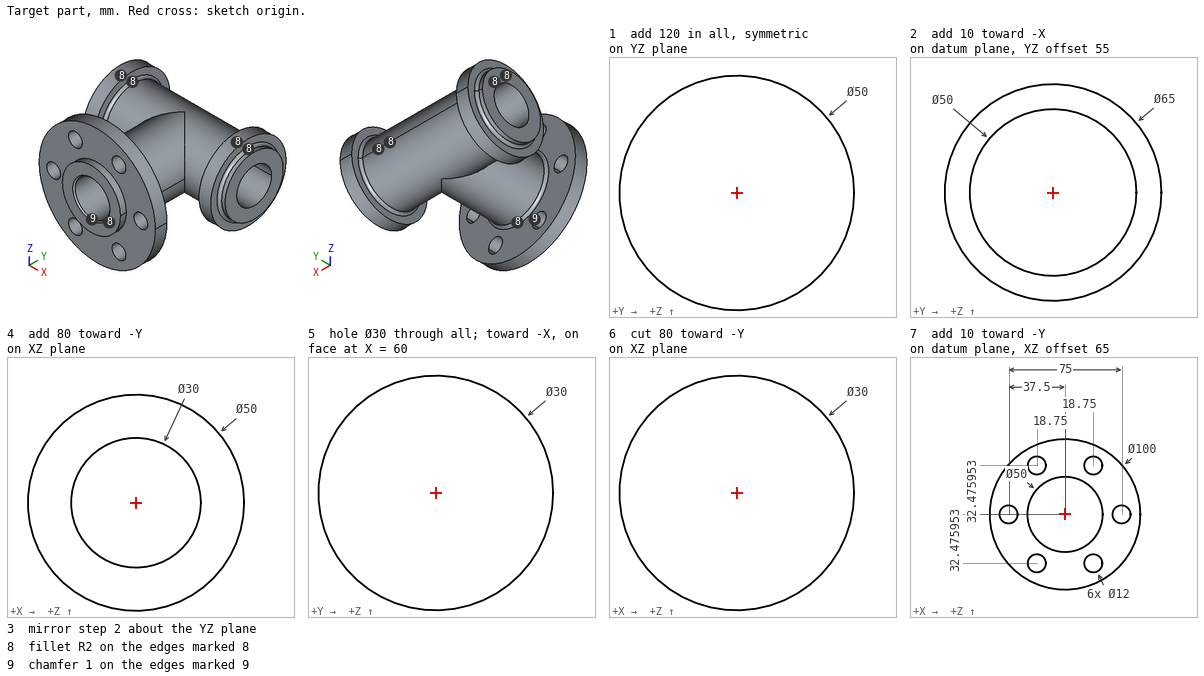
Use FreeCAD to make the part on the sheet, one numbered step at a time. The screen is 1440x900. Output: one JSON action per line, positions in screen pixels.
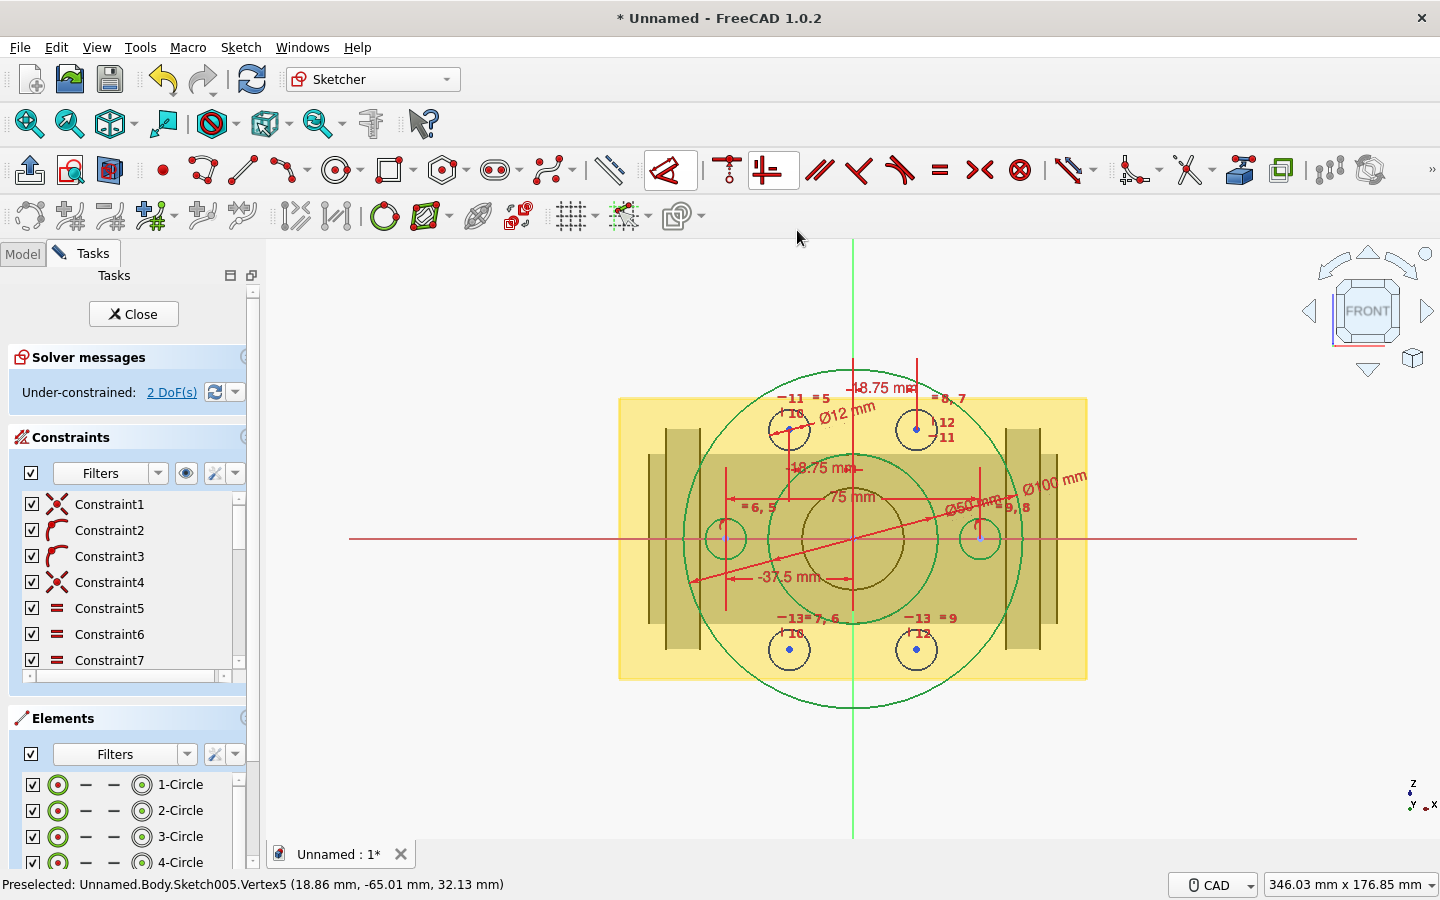
{"action": "left_click", "coordinate": [789, 430]}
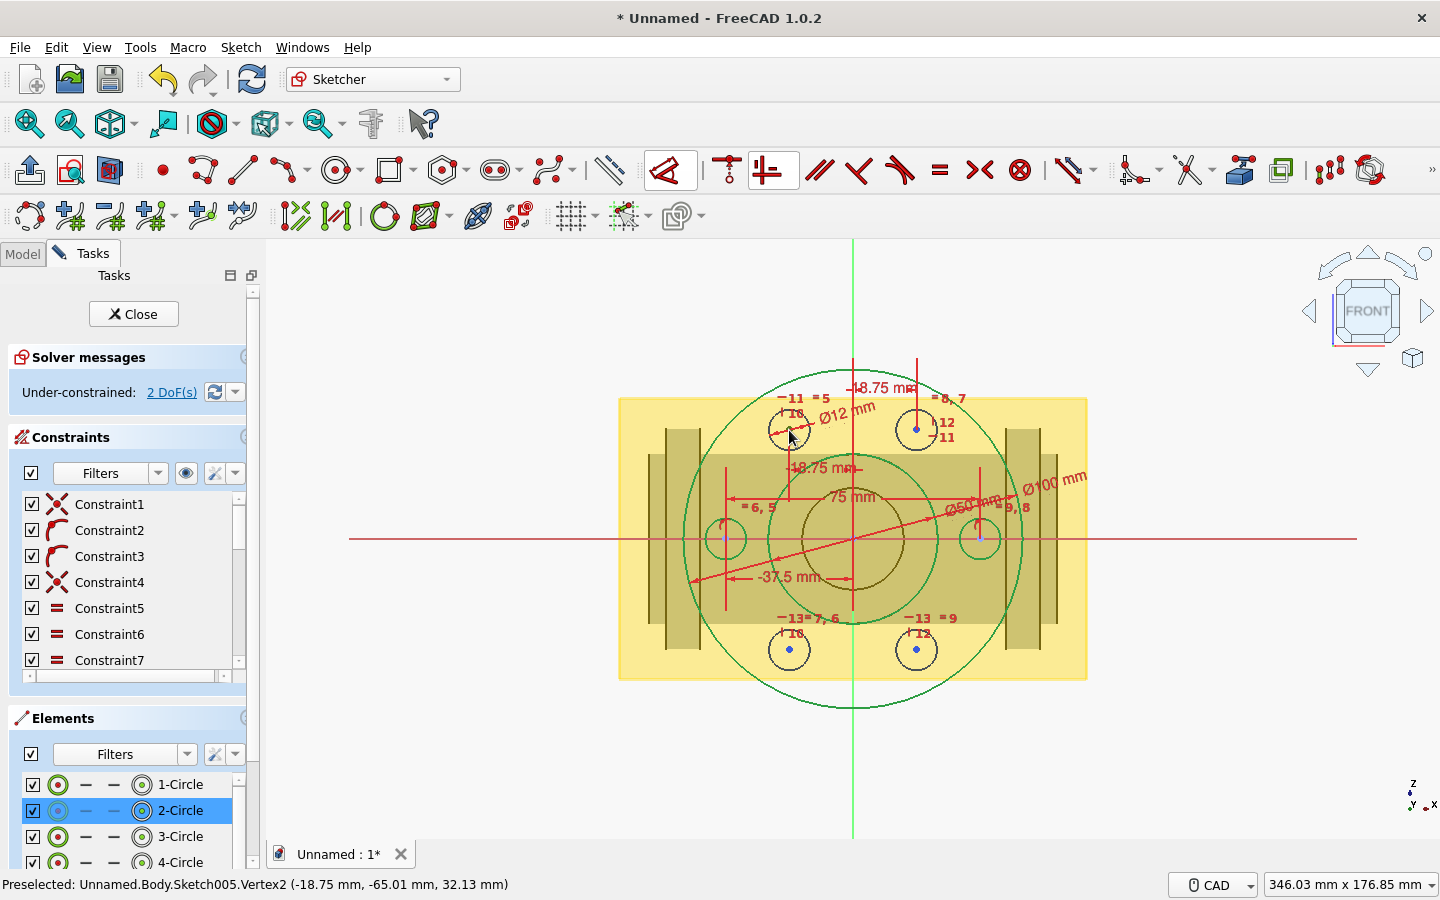
{"action": "key", "text": "i"}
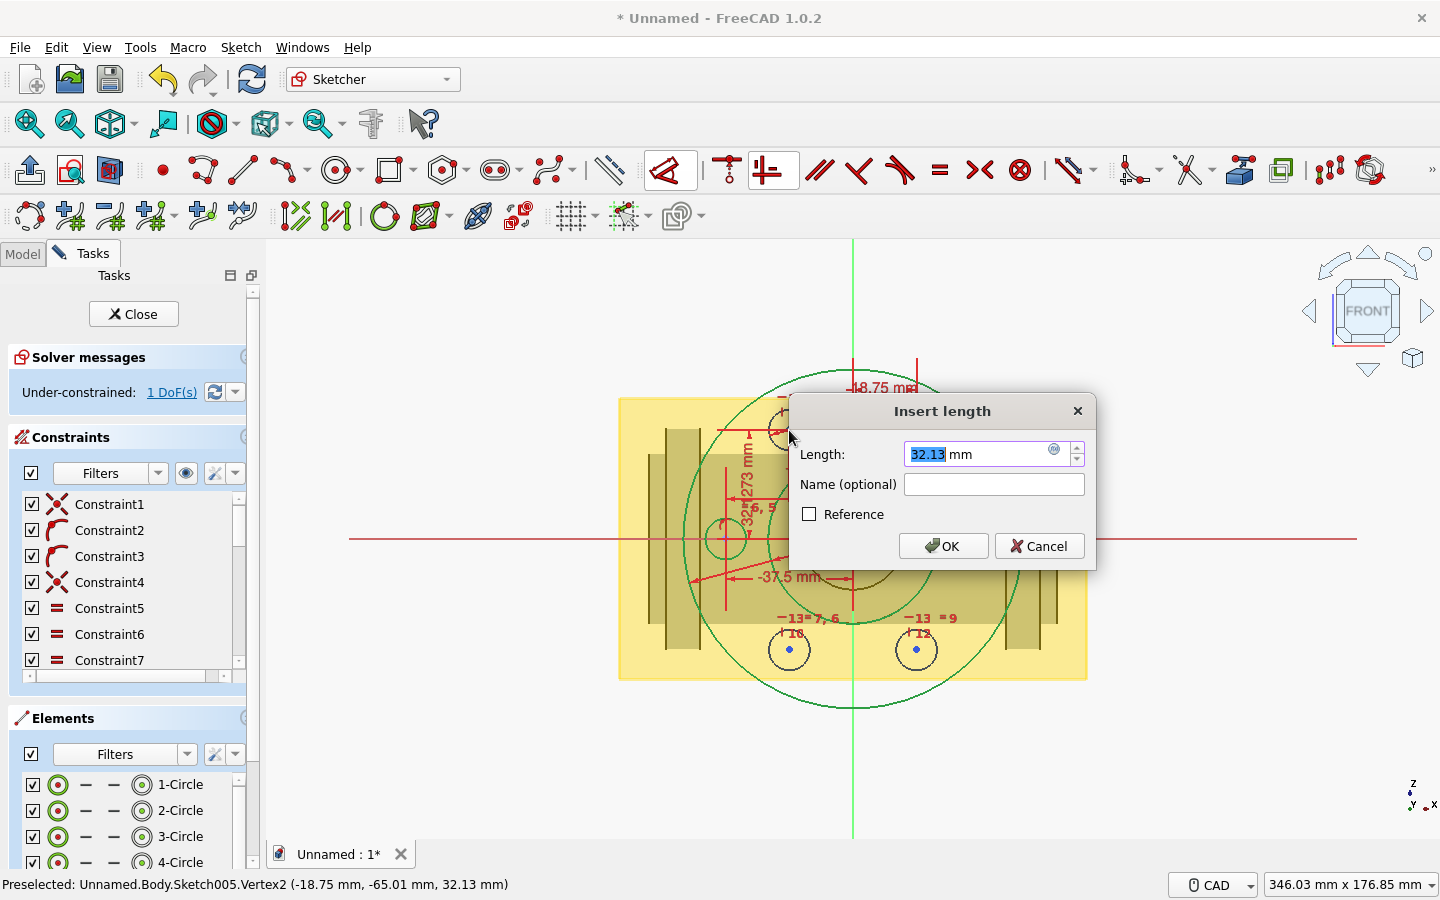
{"action": "type", "text": "32.475953"}
{"action": "key", "text": "Return"}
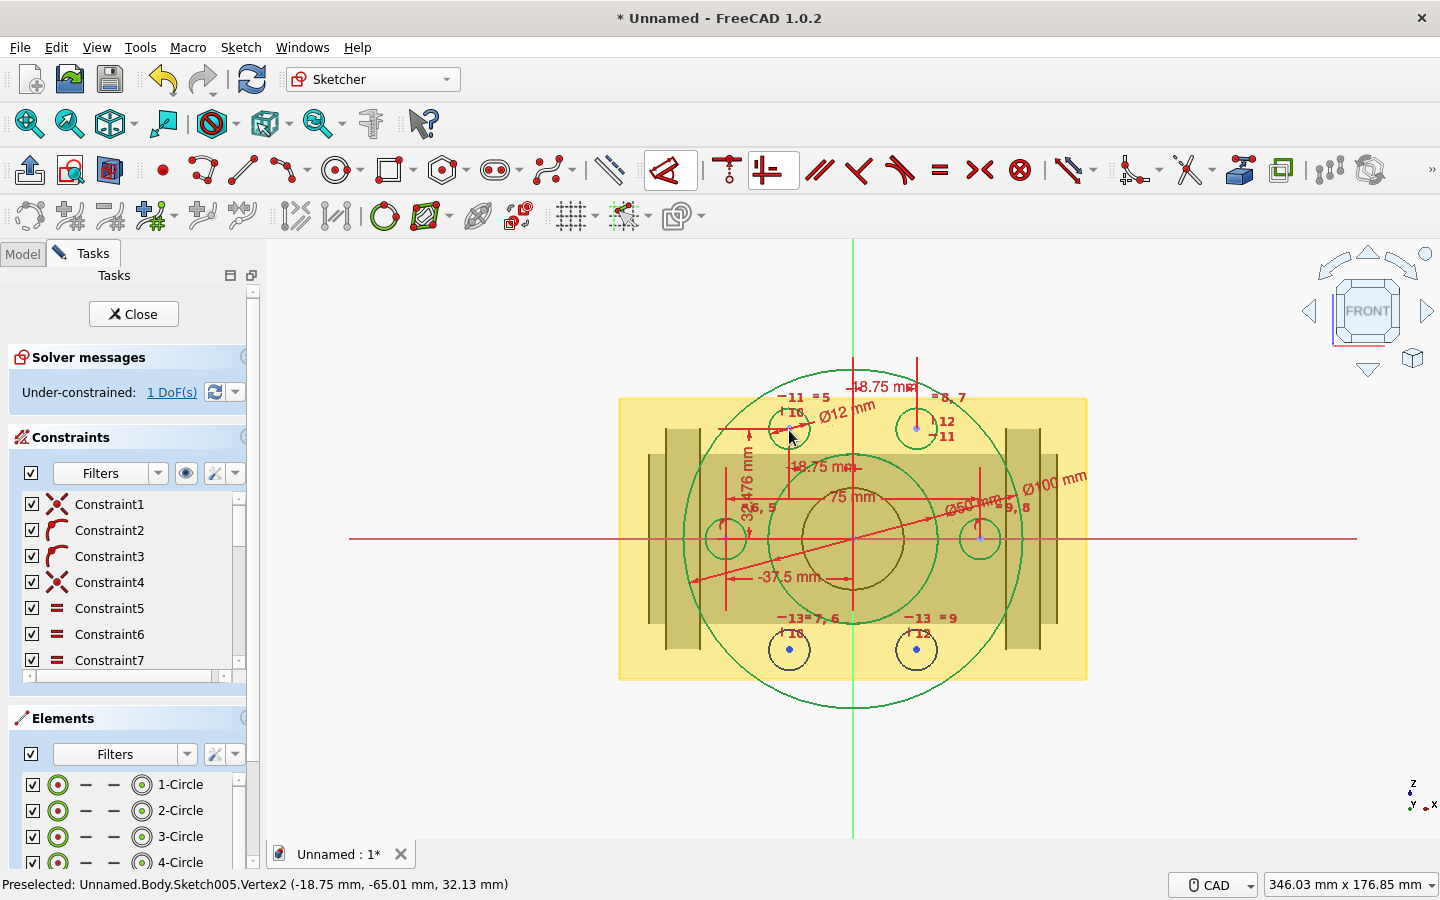
{"action": "left_click", "coordinate": [789, 650]}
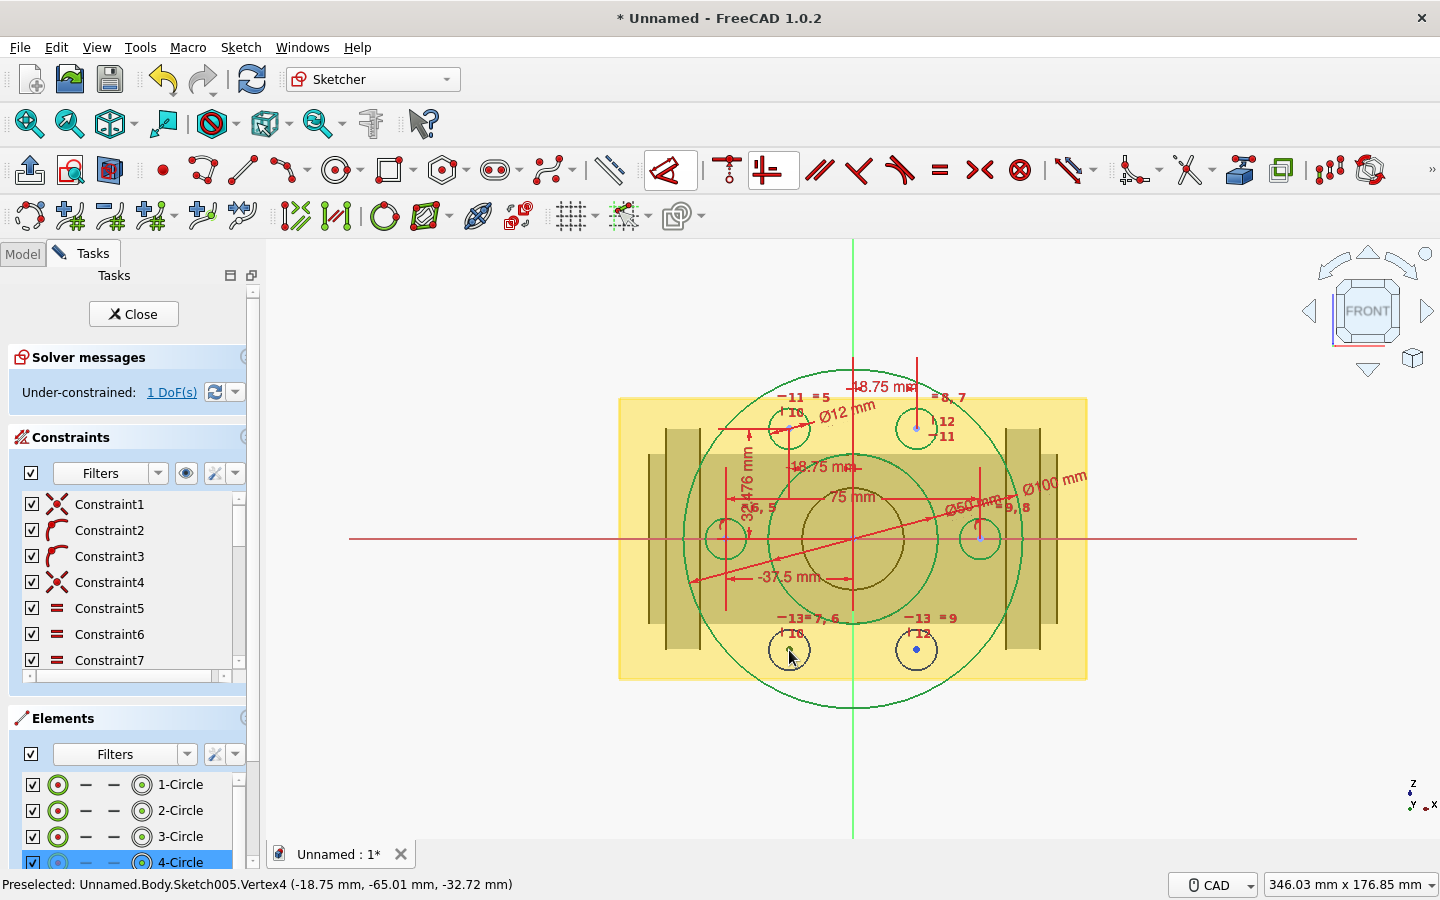
{"action": "key", "text": "i"}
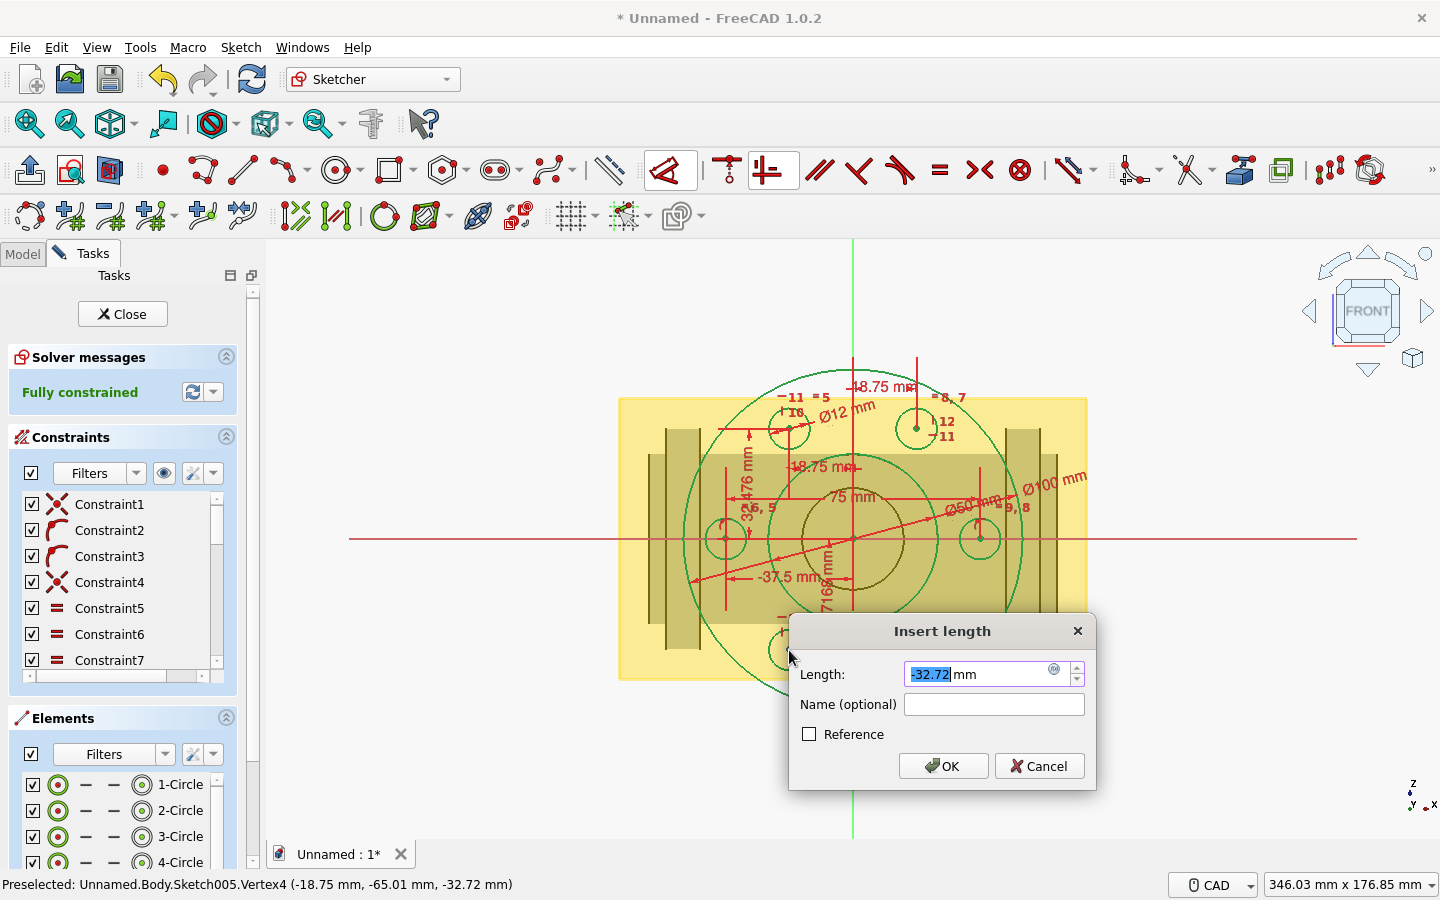
{"action": "type", "text": "-32.475953"}
{"action": "key", "text": "Return"}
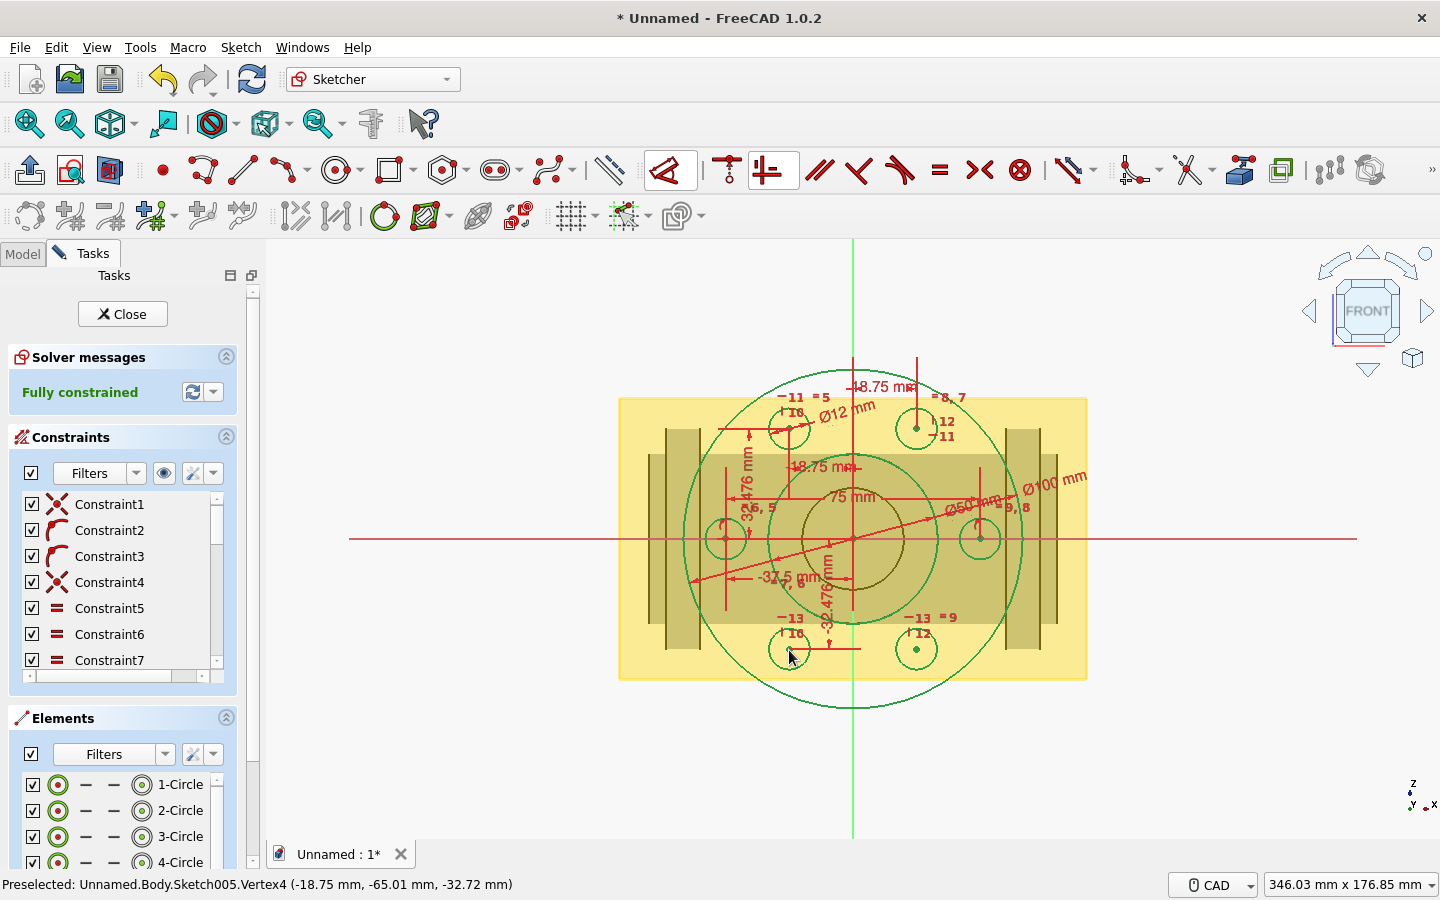
{"action": "left_click", "coordinate": [123, 314]}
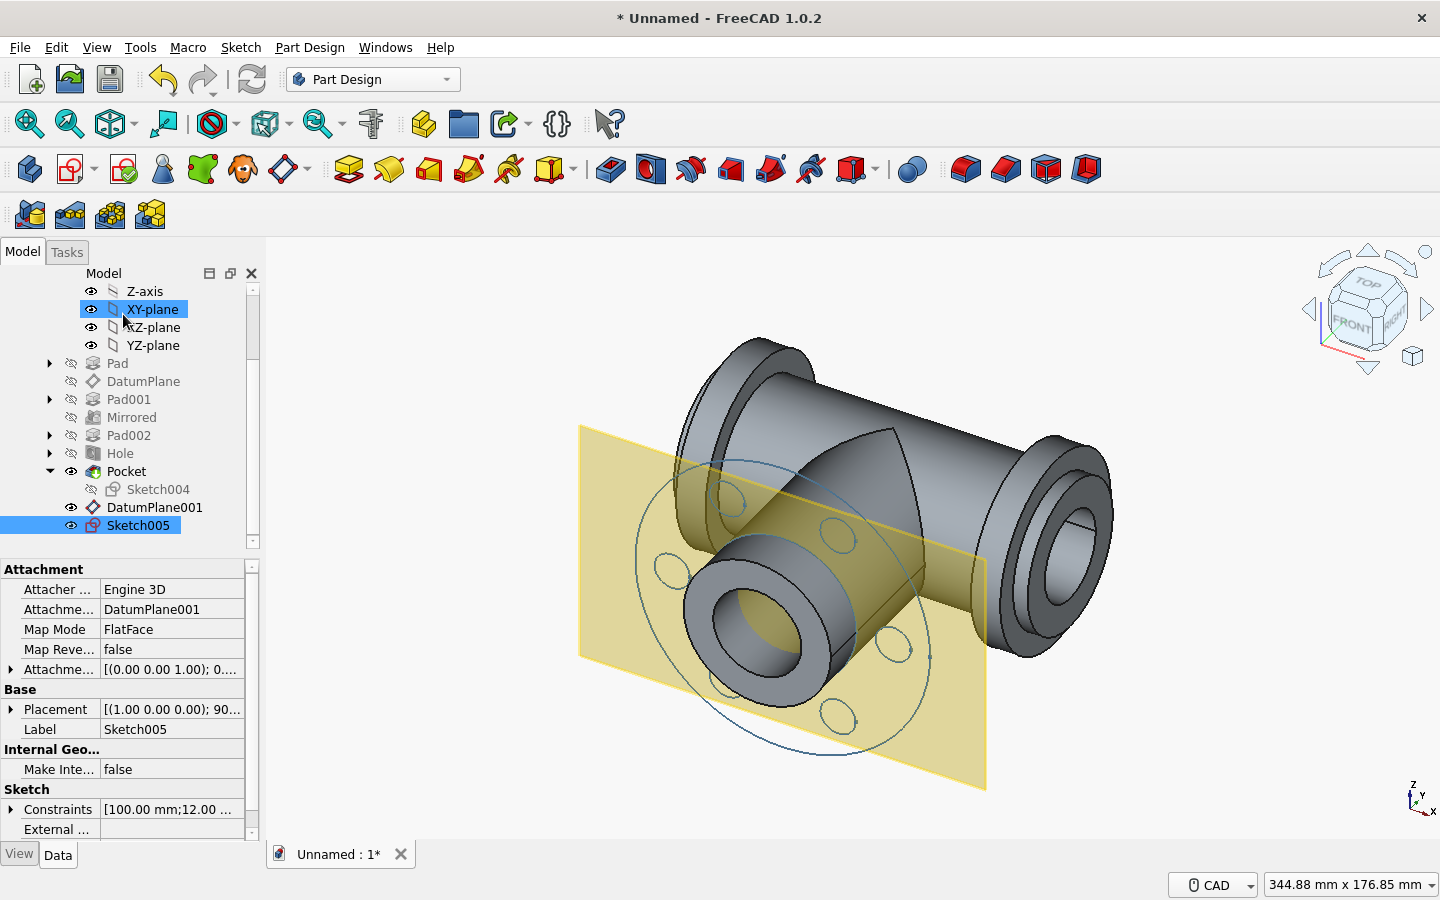
{"action": "left_click", "coordinate": [350, 170]}